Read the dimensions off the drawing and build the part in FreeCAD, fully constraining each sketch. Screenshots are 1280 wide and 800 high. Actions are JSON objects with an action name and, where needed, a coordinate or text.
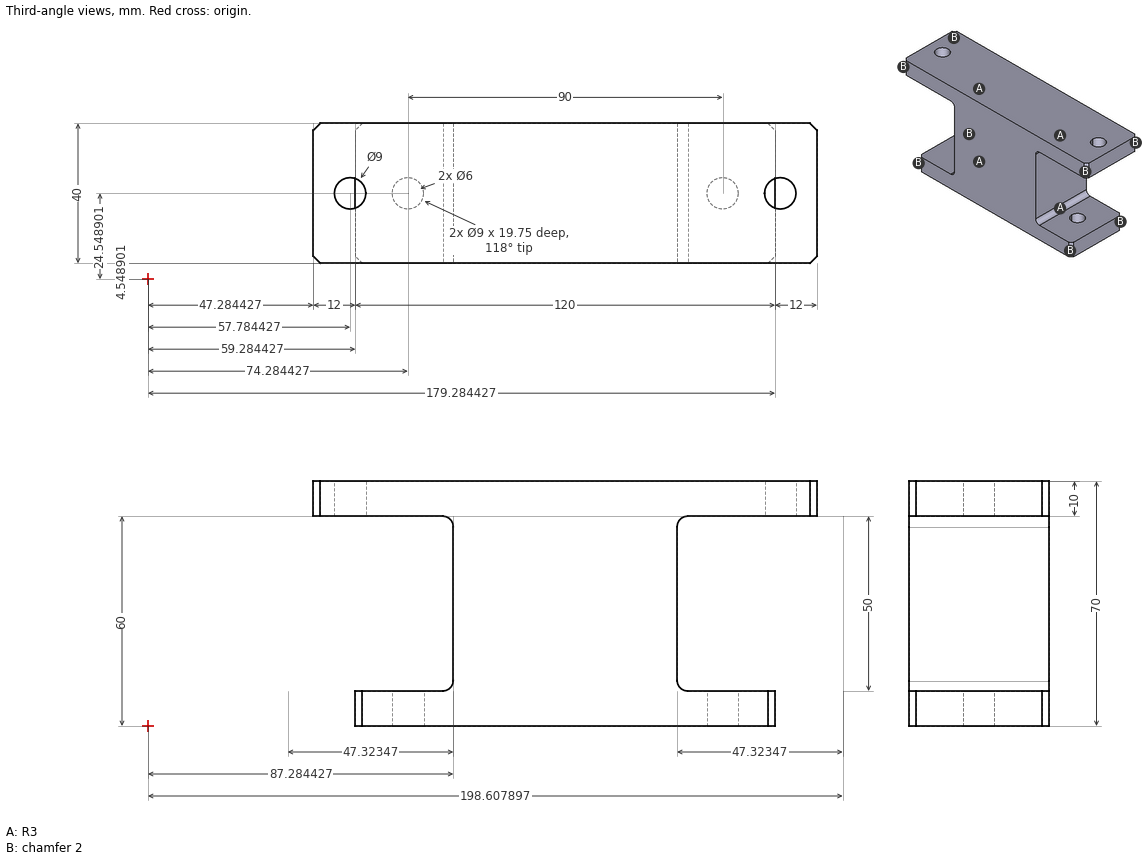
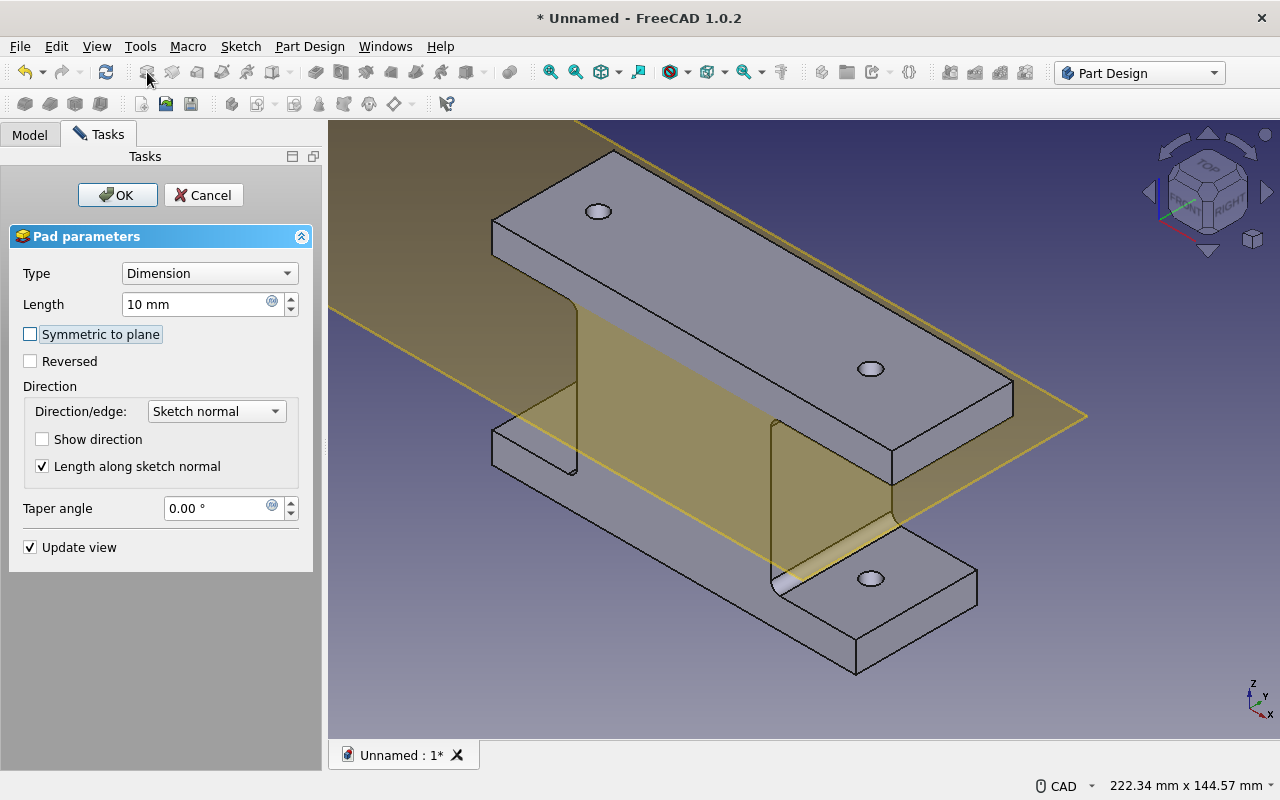
{"action": "left_click", "coordinate": [118, 195]}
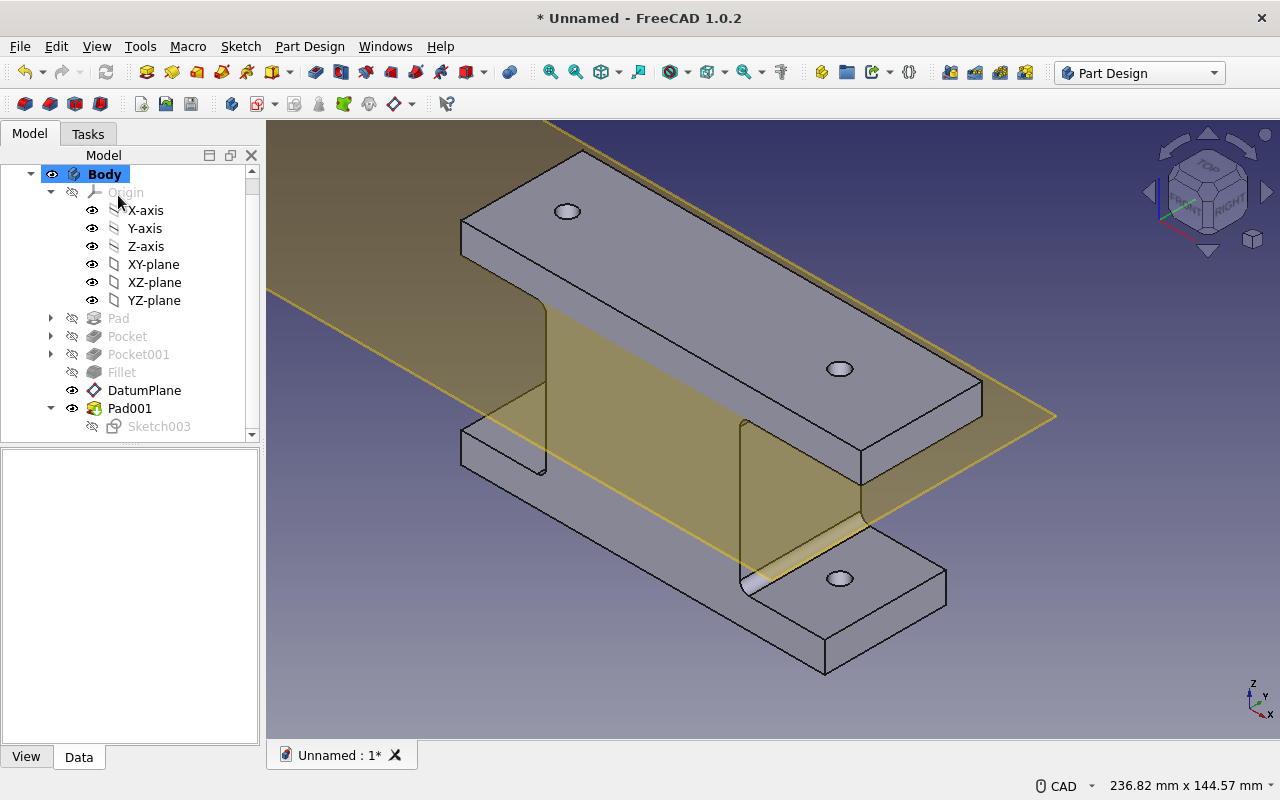
{"action": "left_click", "coordinate": [117, 390]}
{"action": "key", "text": "space"}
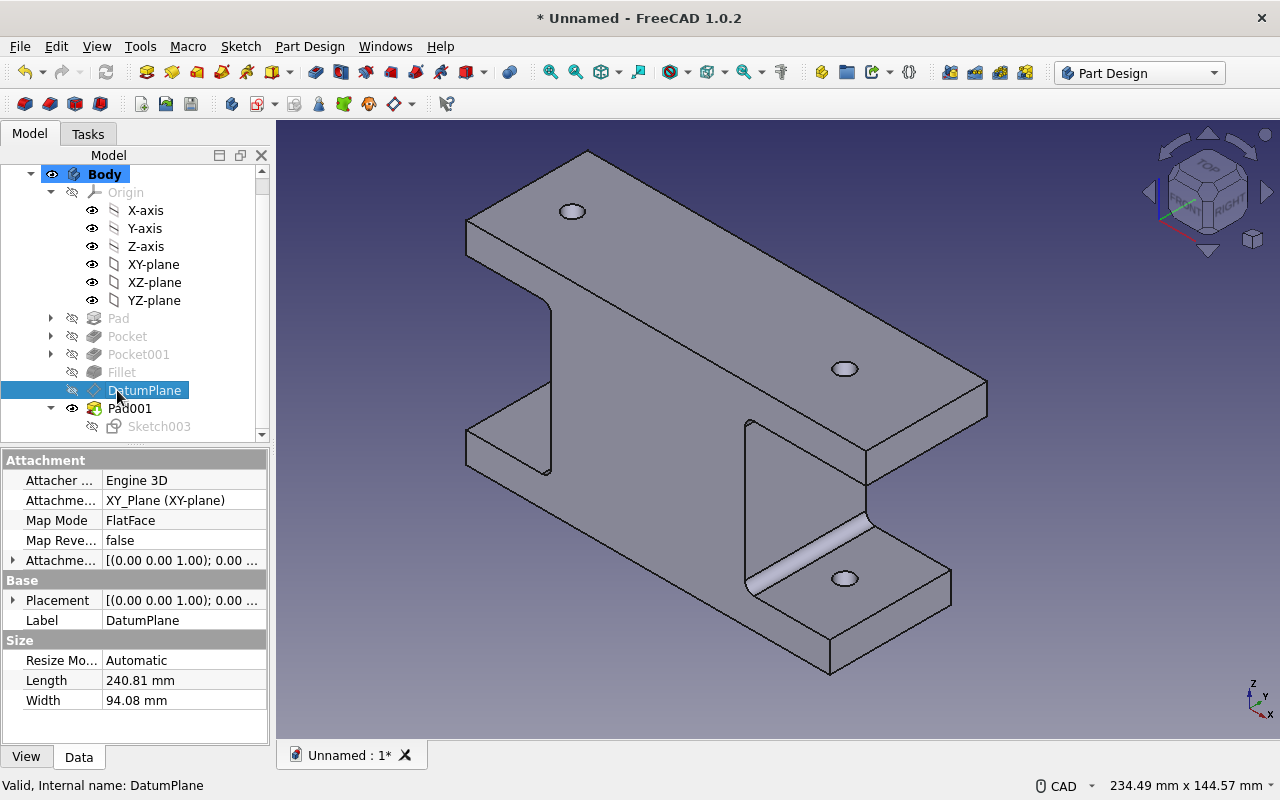
{"action": "left_click", "coordinate": [727, 300]}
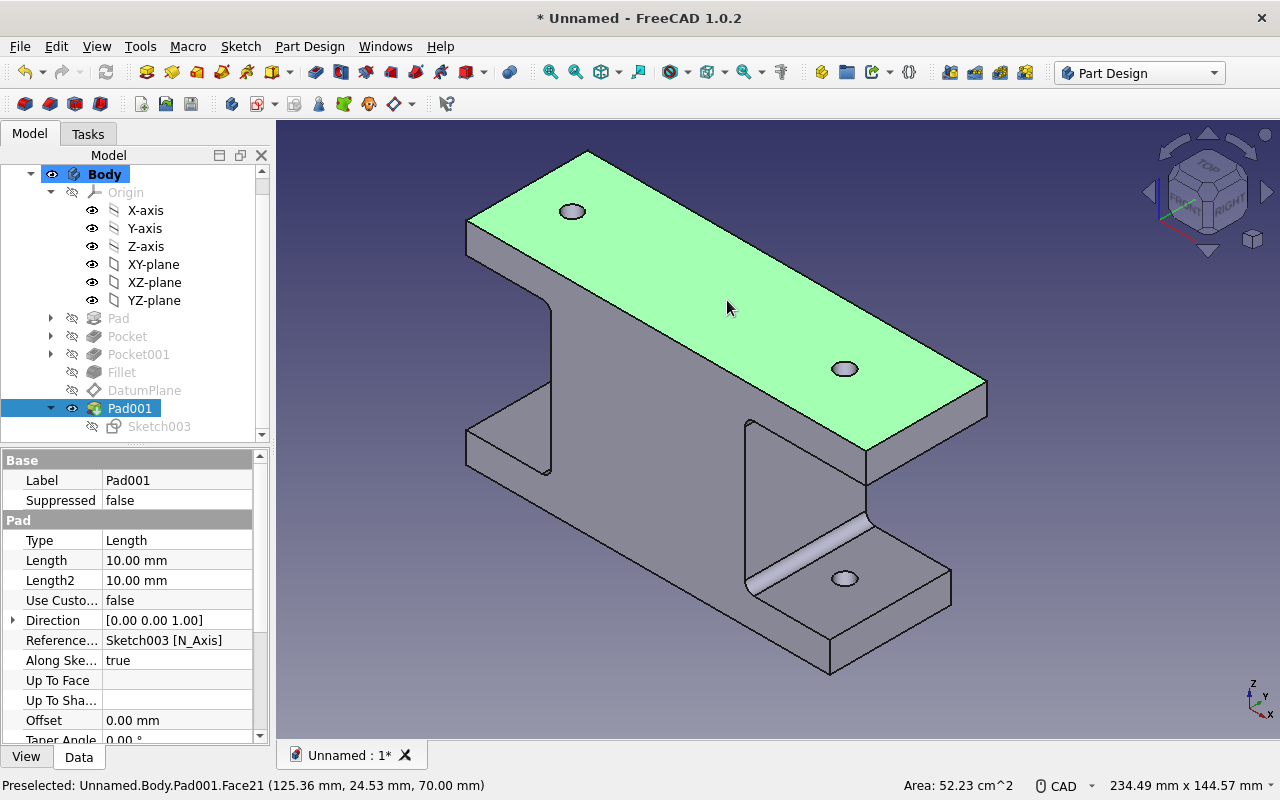
{"action": "left_click", "coordinate": [256, 104]}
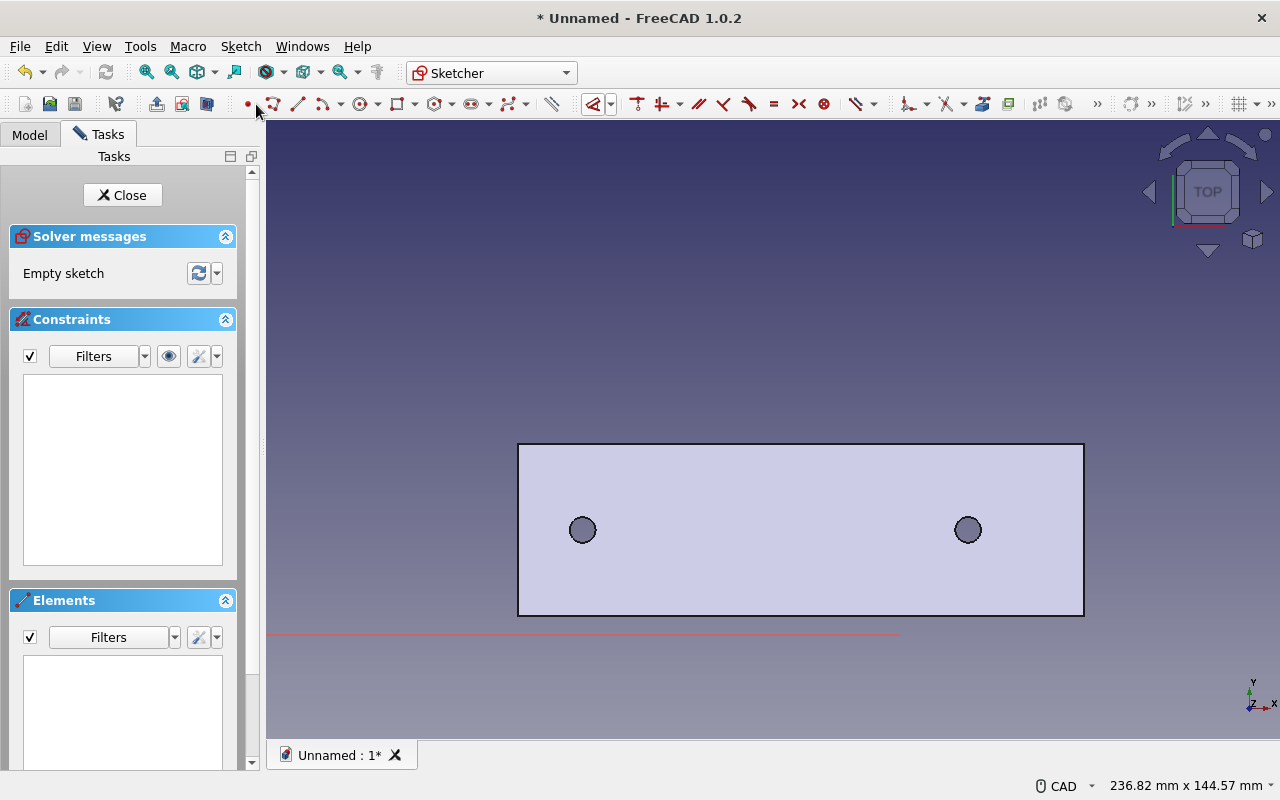
{"action": "scroll", "coordinate": [704, 430], "scroll_direction": "down", "scroll_amount": 5}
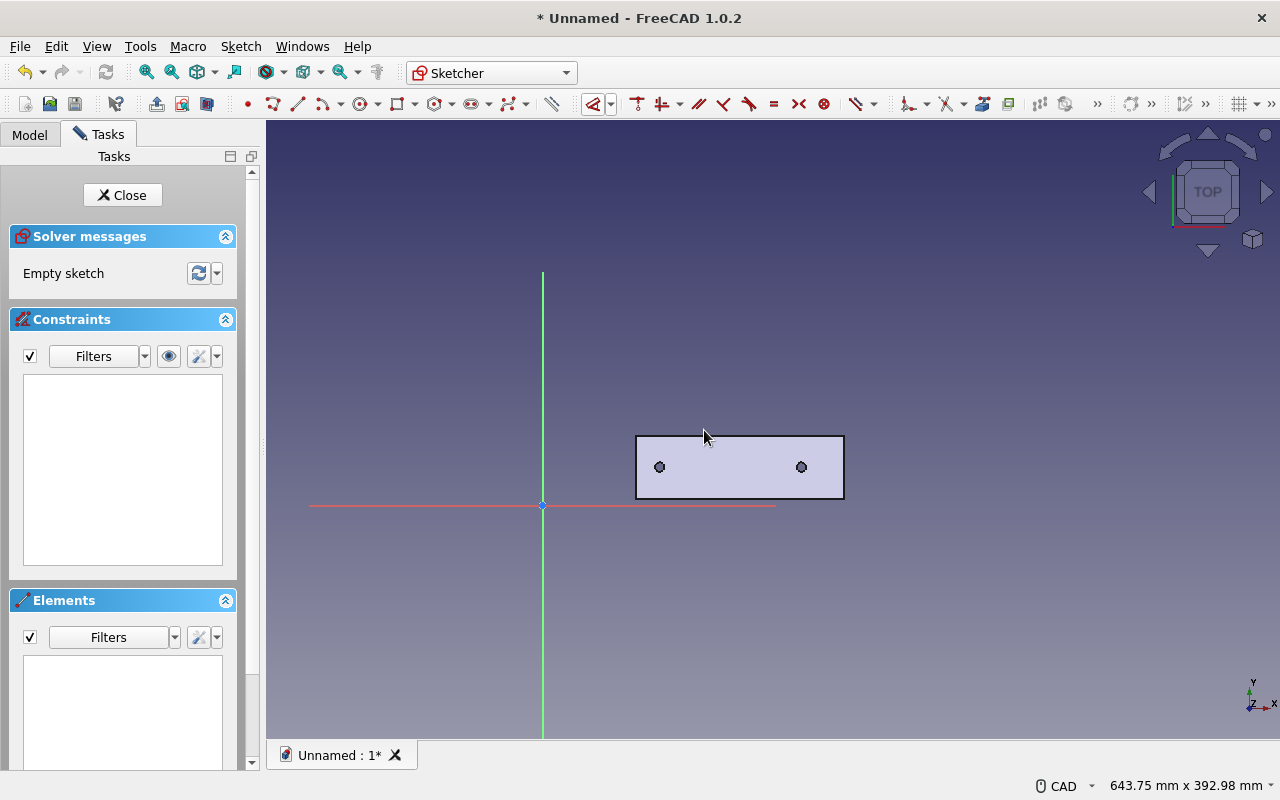
{"action": "scroll", "coordinate": [567, 479], "scroll_direction": "up", "scroll_amount": 9}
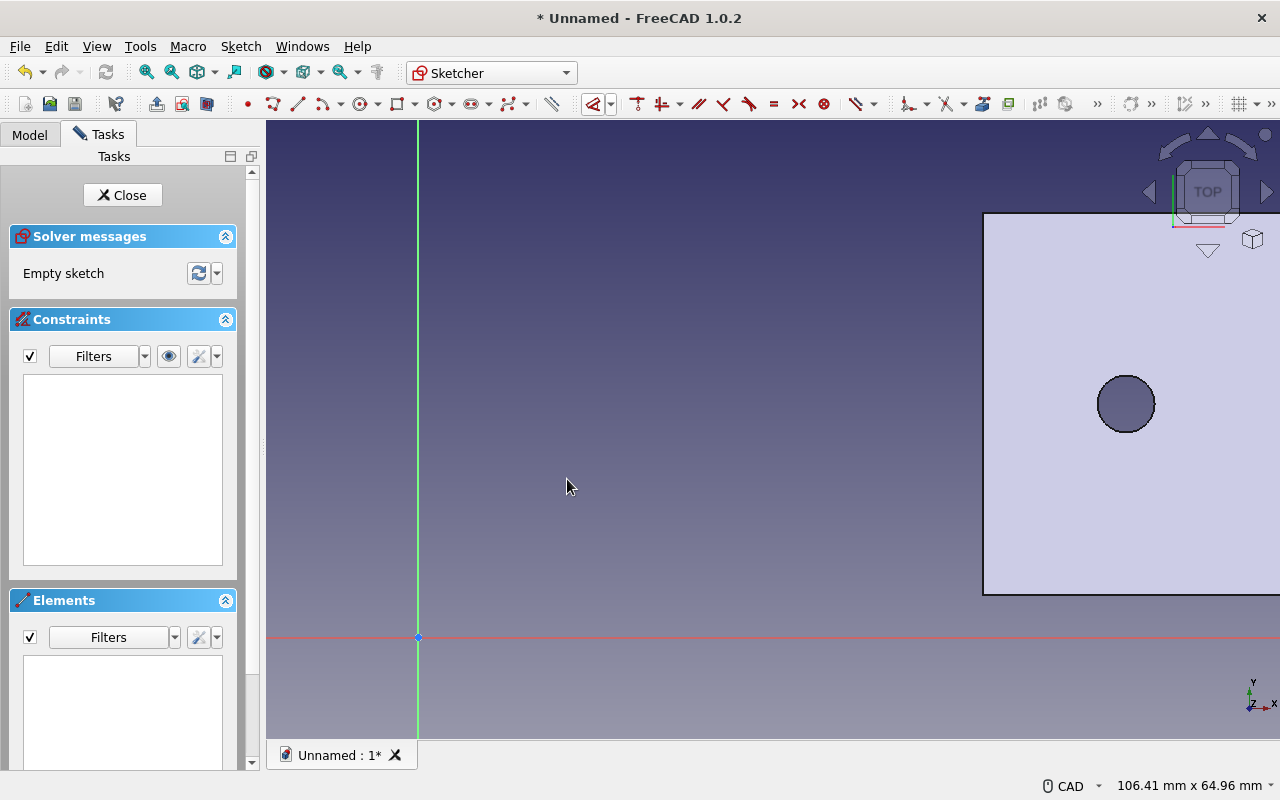
{"action": "key", "text": "g r"}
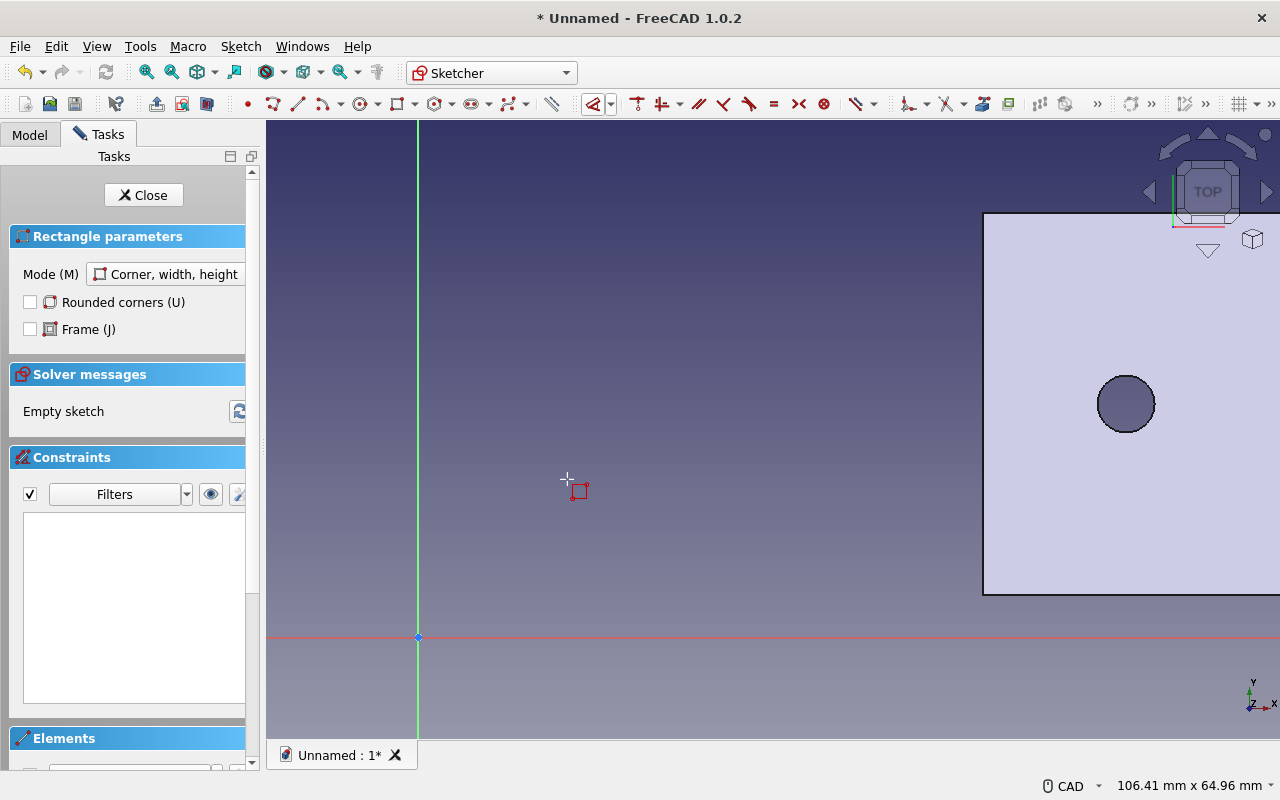
{"action": "left_click", "coordinate": [869, 213]}
{"action": "left_click", "coordinate": [983, 595]}
{"action": "key", "text": "Escape"}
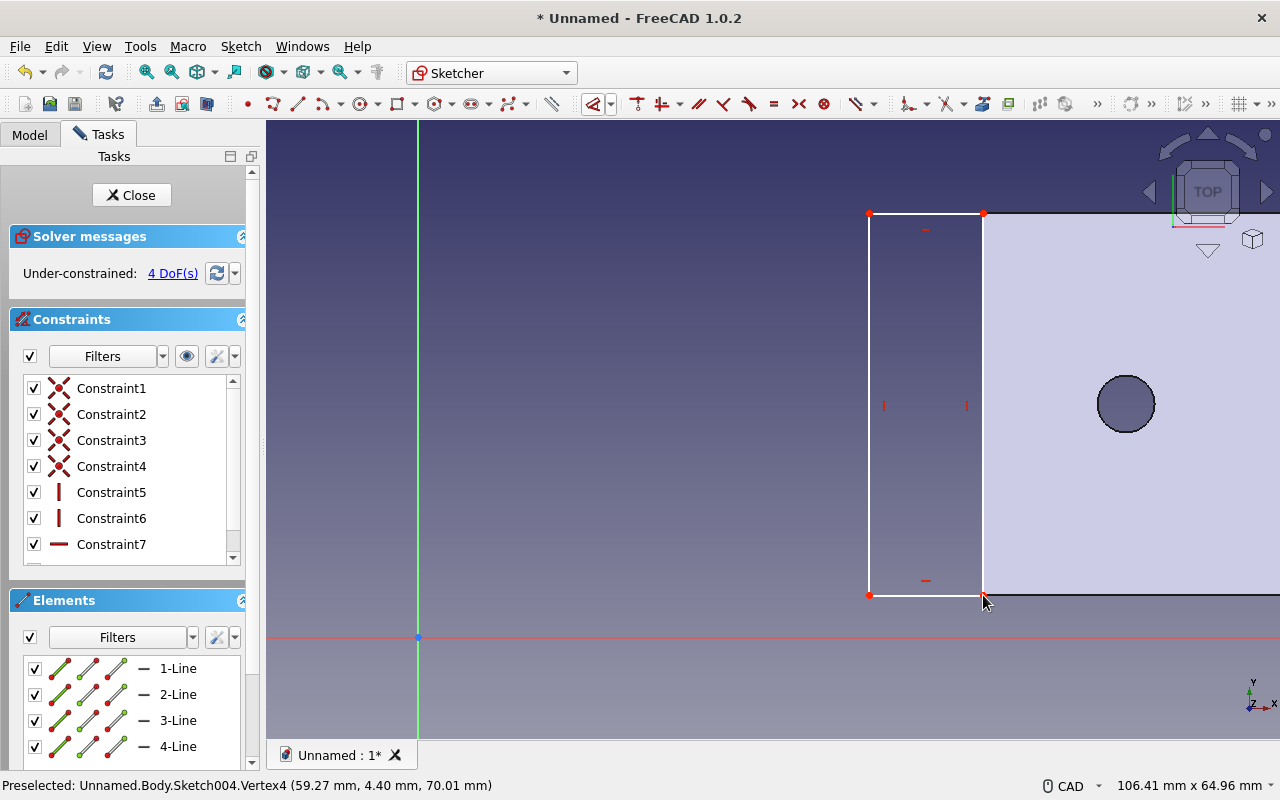
{"action": "left_click", "coordinate": [869, 329]}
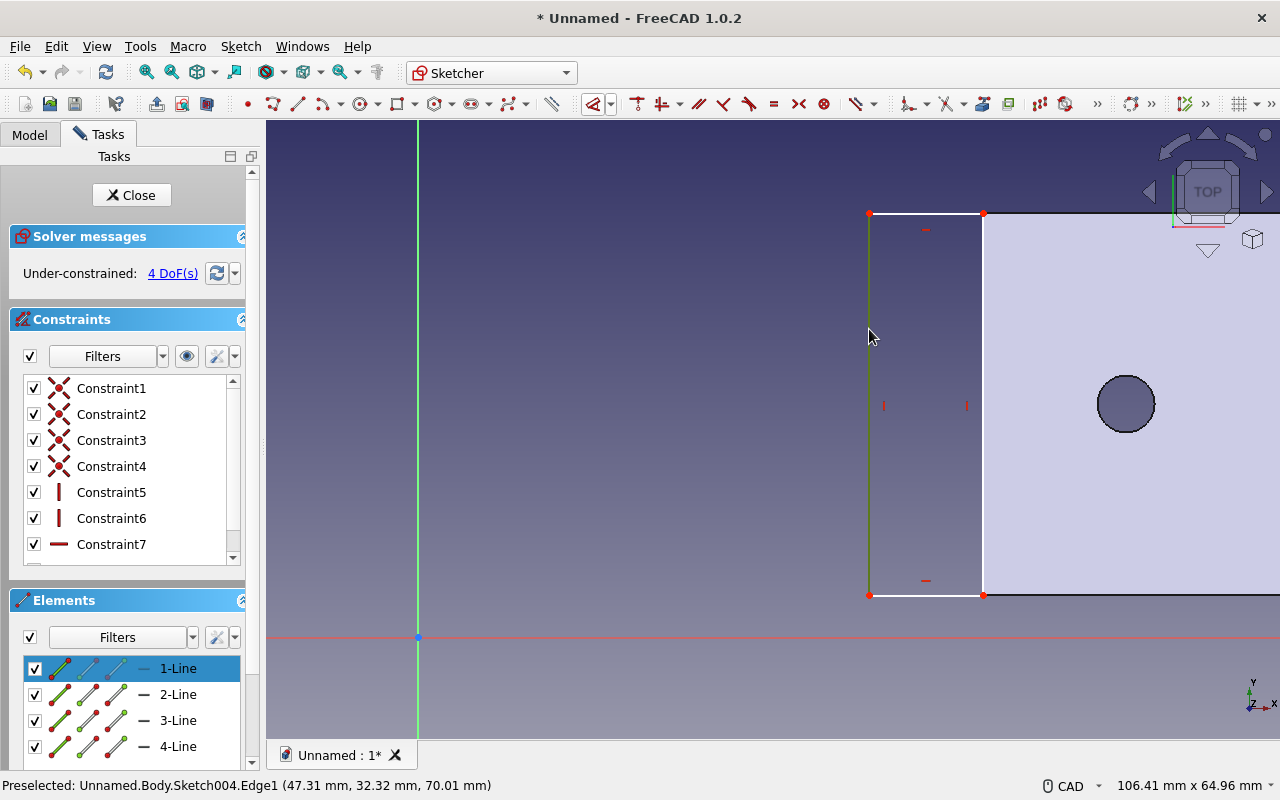
{"action": "key", "text": "i"}